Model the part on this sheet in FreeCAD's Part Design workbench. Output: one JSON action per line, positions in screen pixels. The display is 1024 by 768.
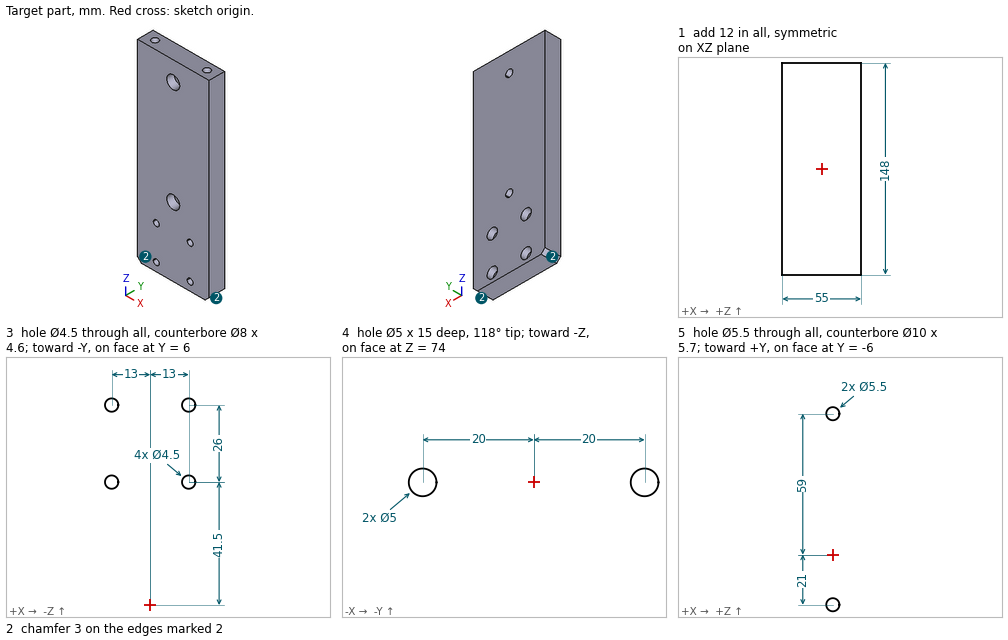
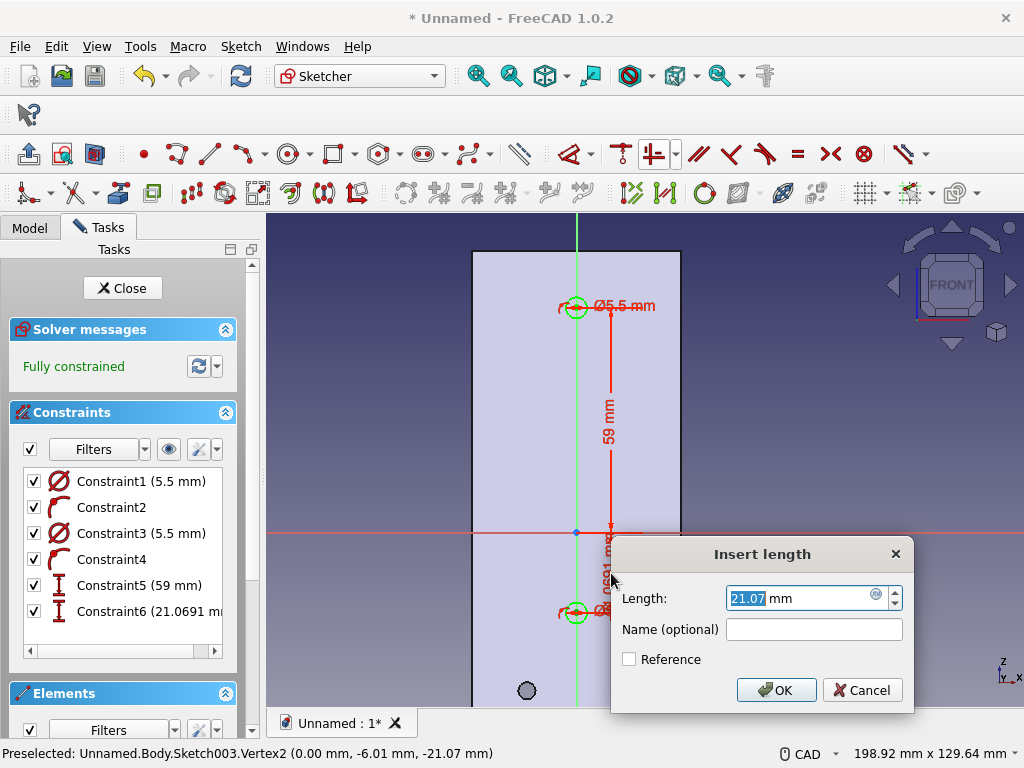
{"action": "type", "text": "21"}
{"action": "key", "text": "Return"}
{"action": "key", "text": "Escape"}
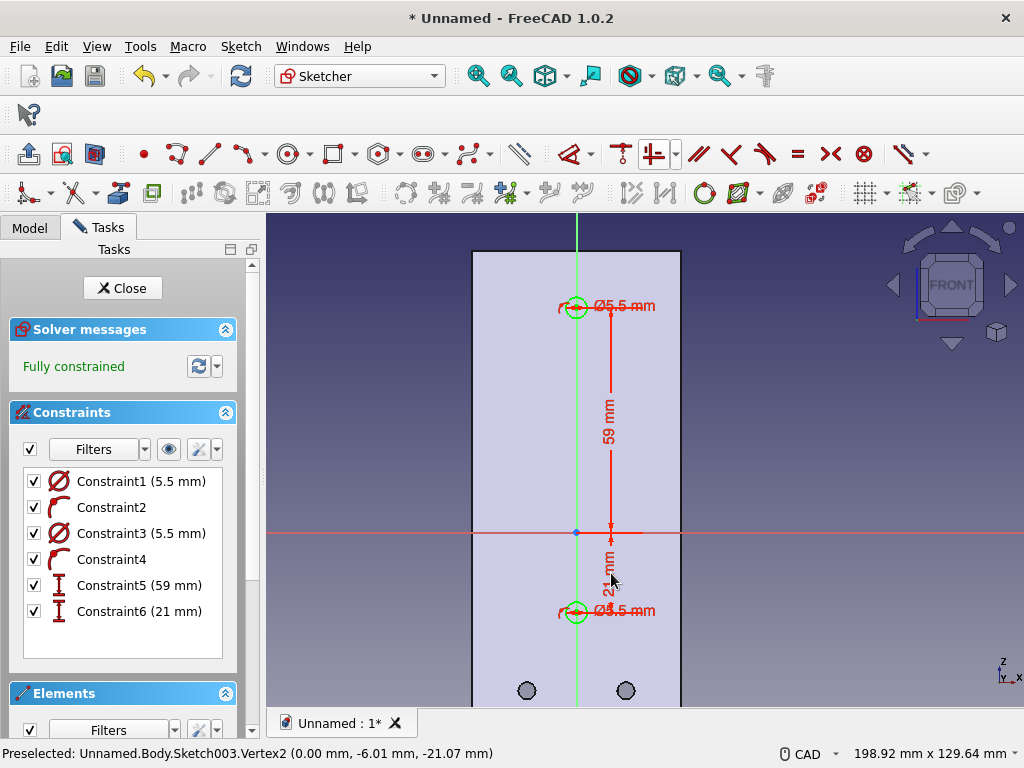
{"action": "left_click", "coordinate": [123, 288]}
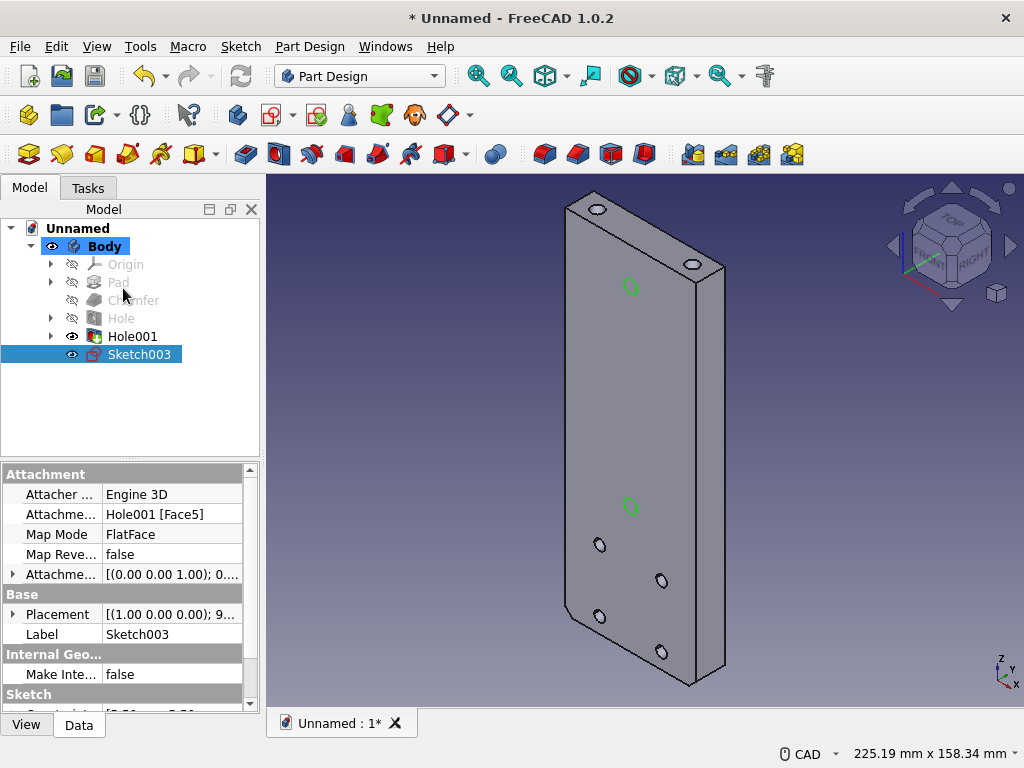
{"action": "left_click", "coordinate": [279, 154]}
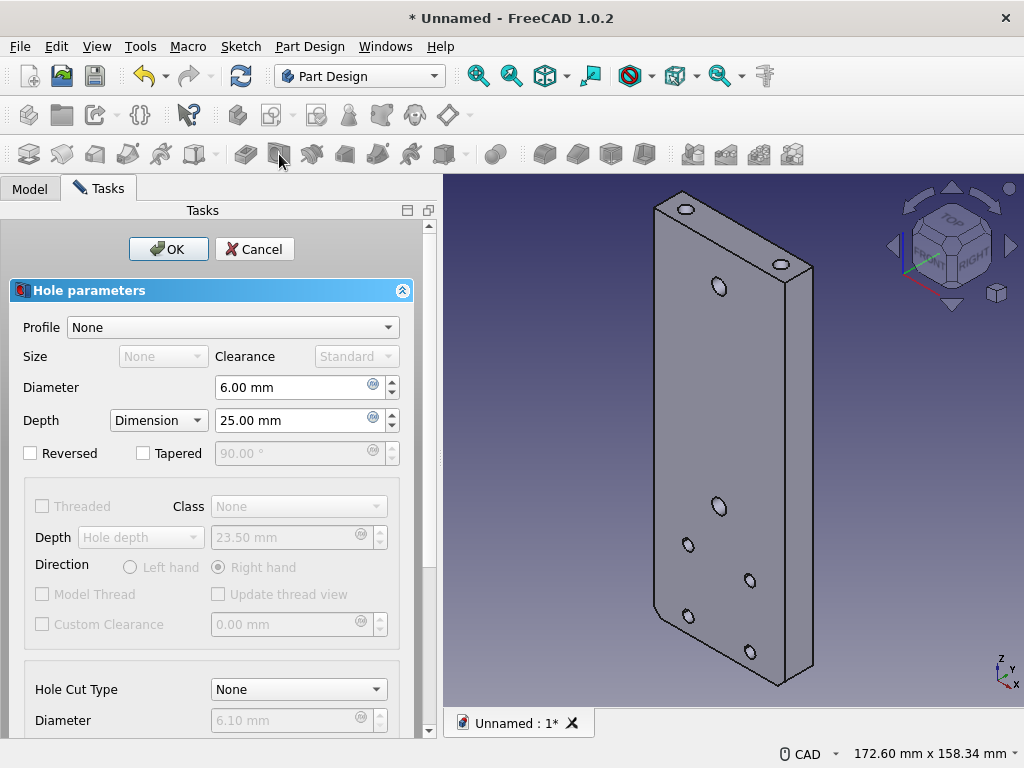
{"action": "triple_click", "coordinate": [300, 388]}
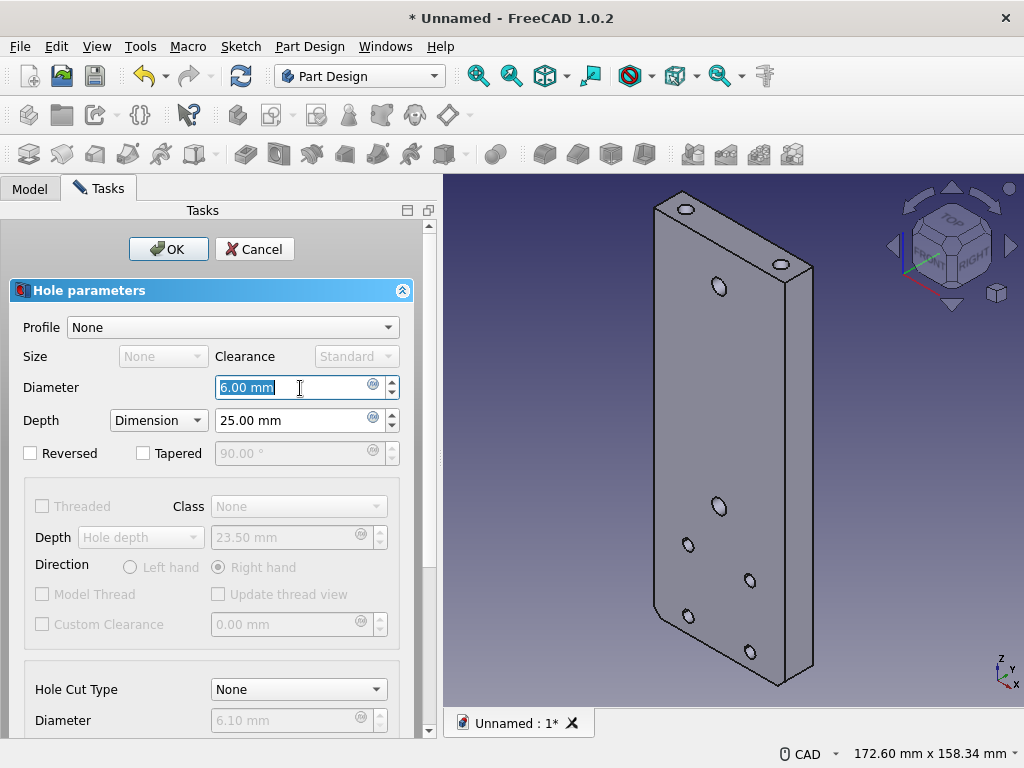
{"action": "type", "text": "5.5"}
{"action": "key", "text": "Tab"}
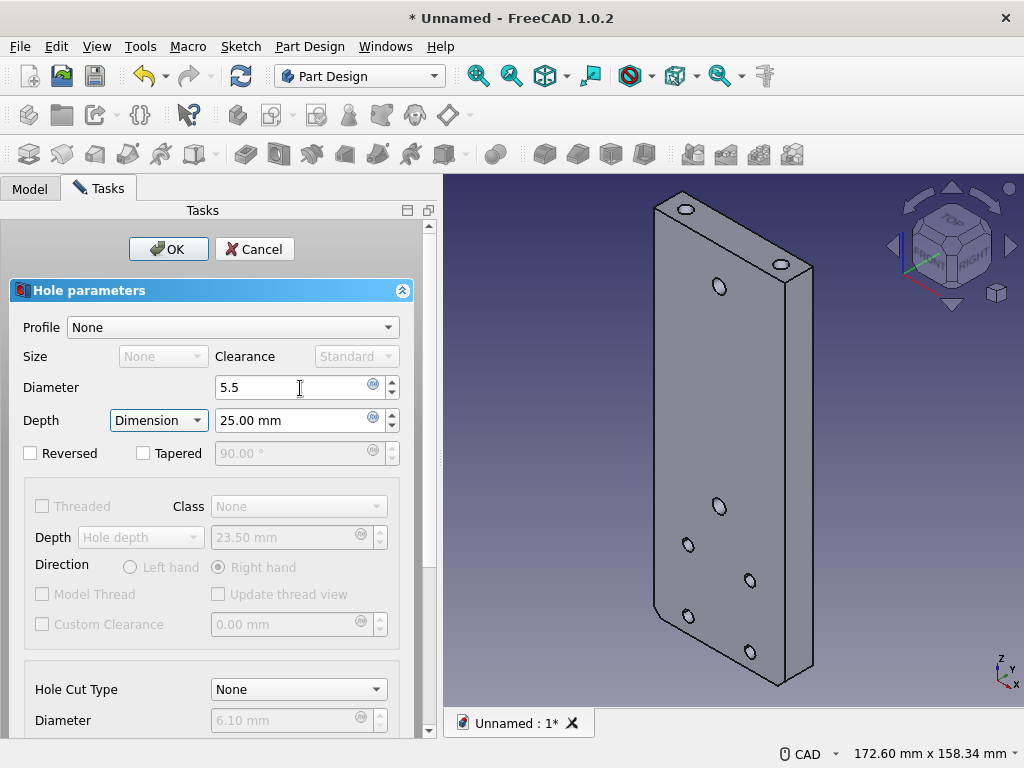
{"action": "left_click", "coordinate": [160, 420]}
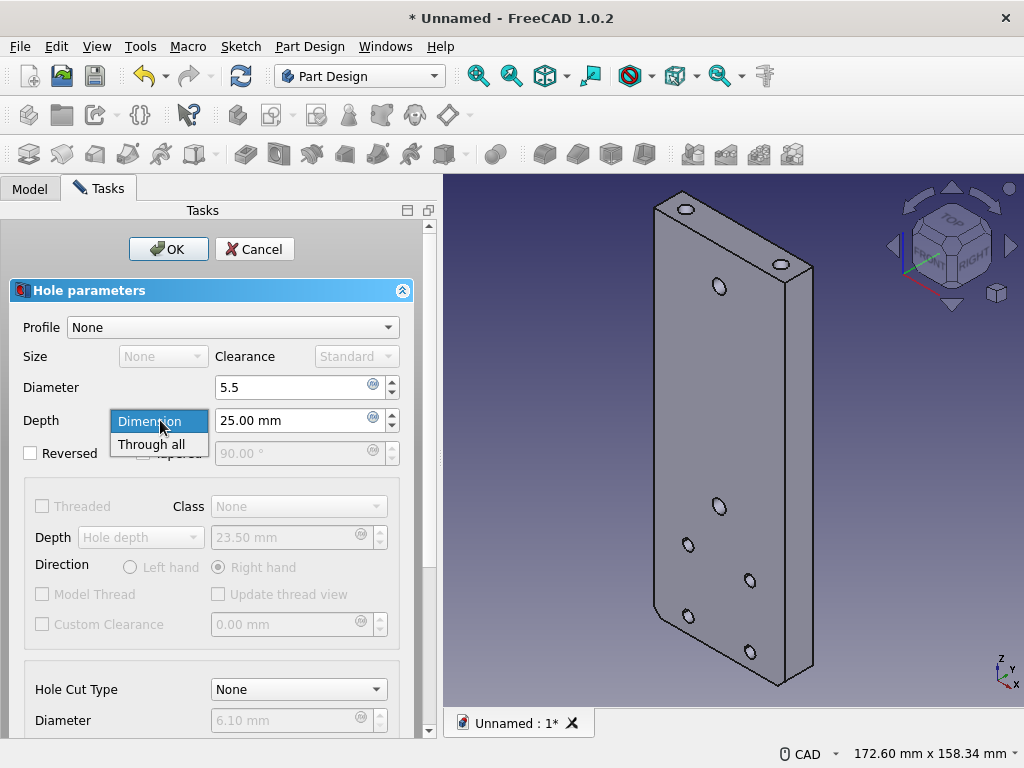
{"action": "left_click", "coordinate": [158, 444]}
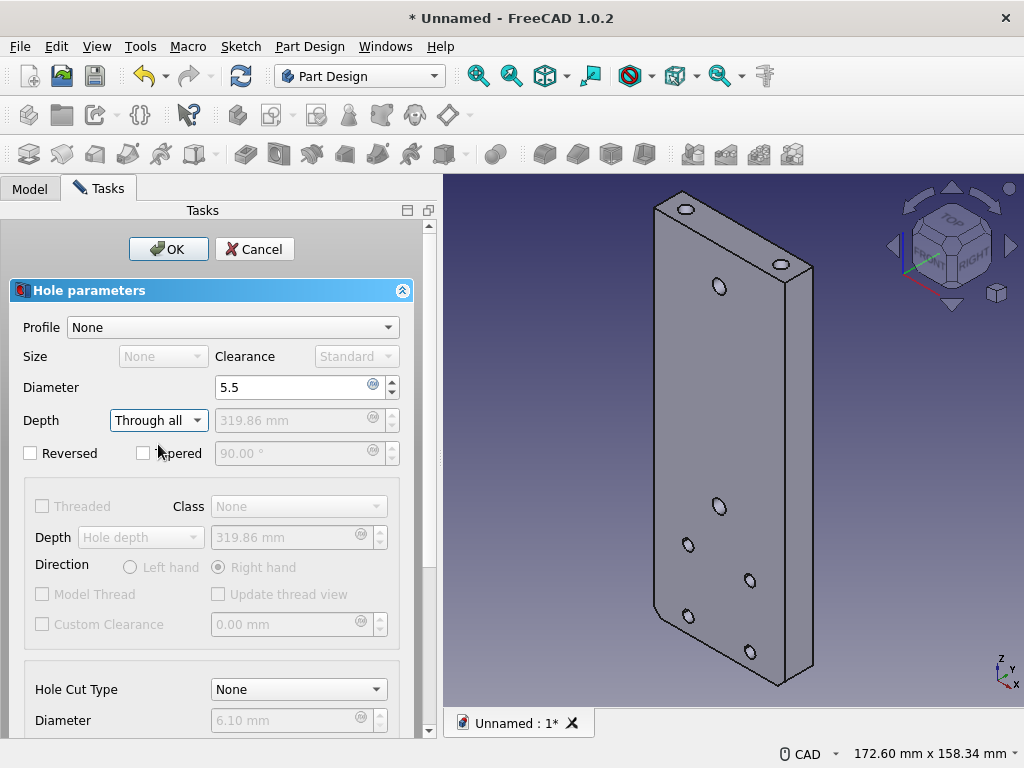
{"action": "left_click", "coordinate": [300, 690]}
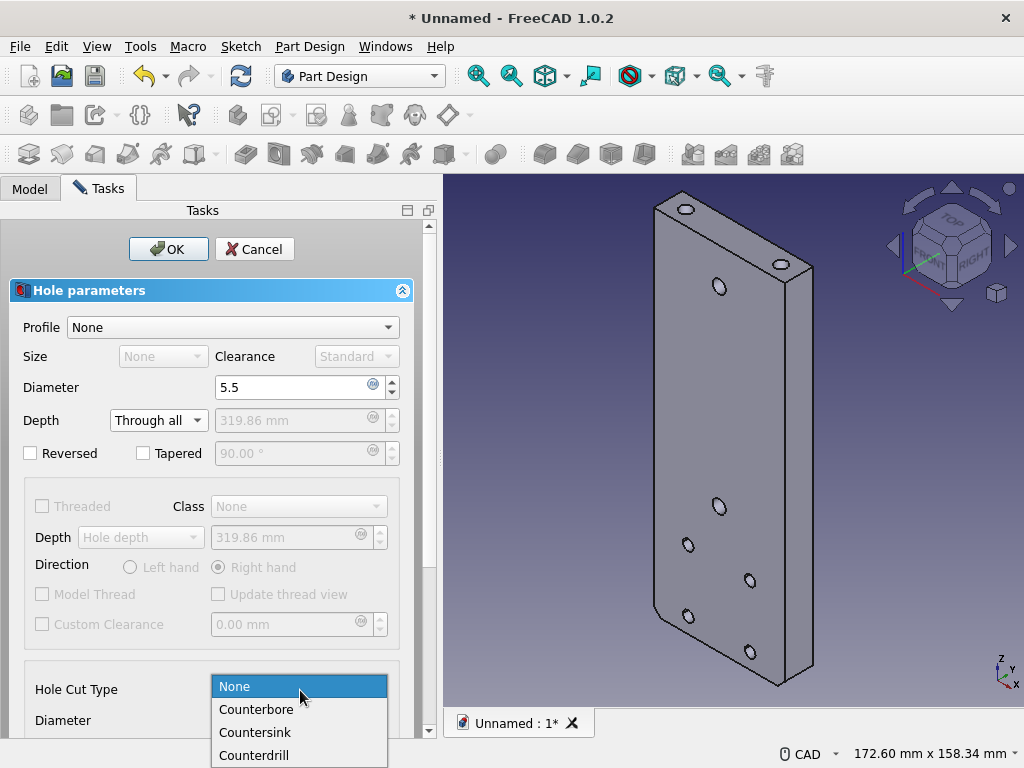
{"action": "left_click", "coordinate": [298, 710]}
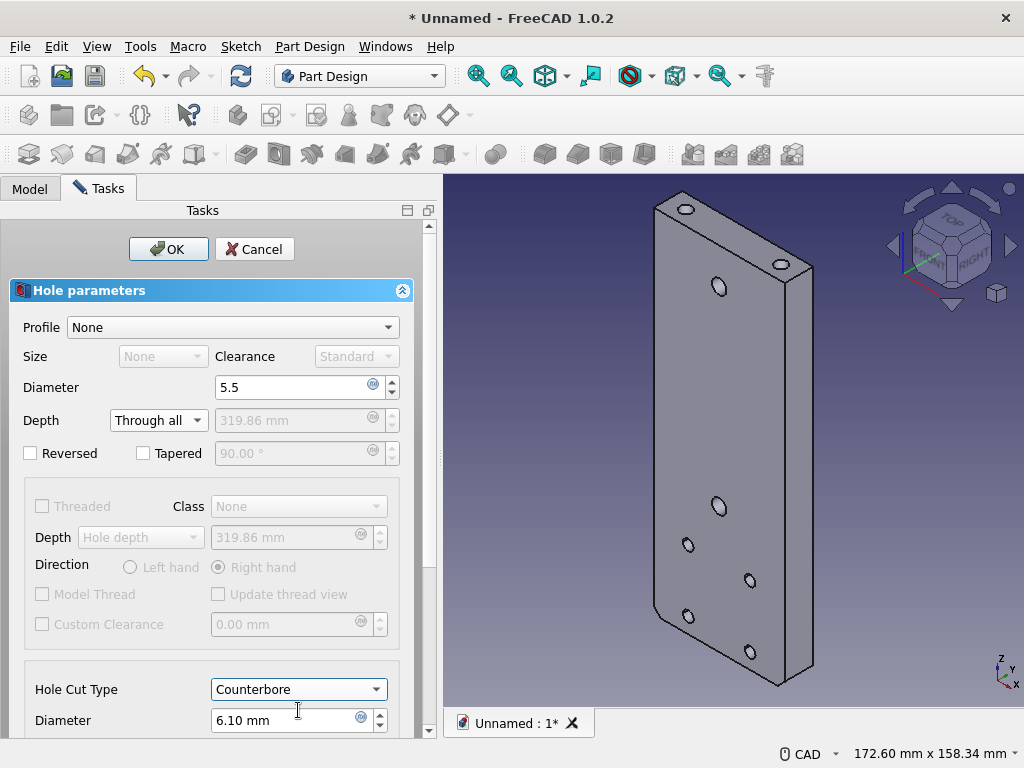
{"action": "triple_click", "coordinate": [292, 720]}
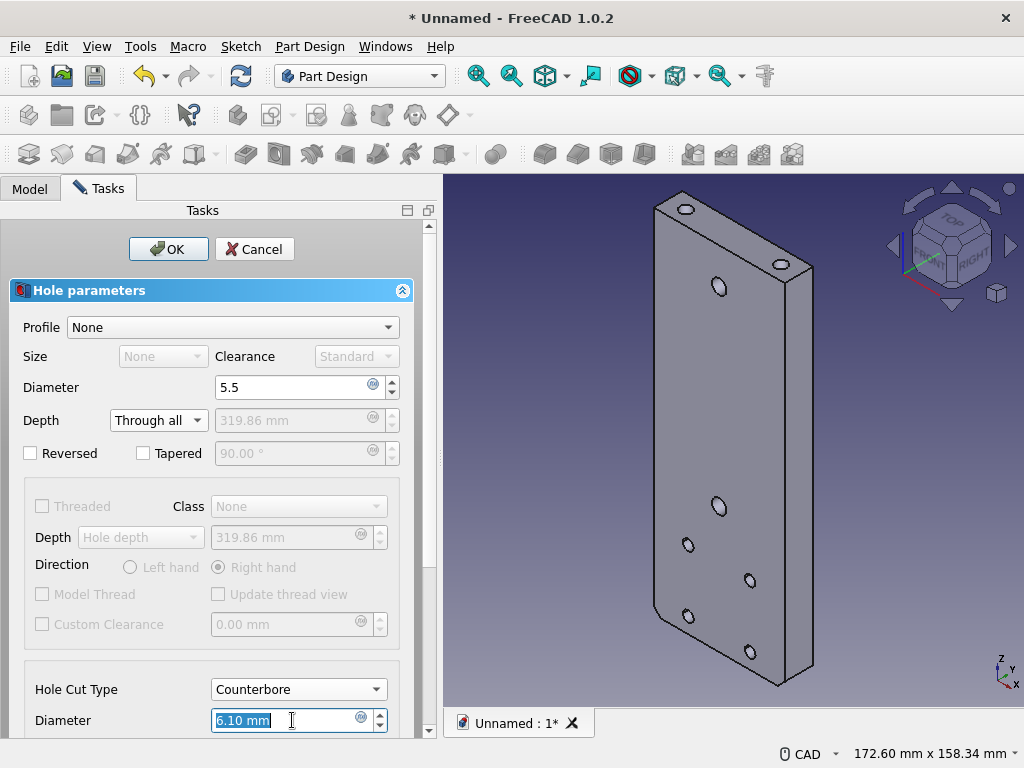
{"action": "type", "text": "10"}
{"action": "key", "text": "Tab"}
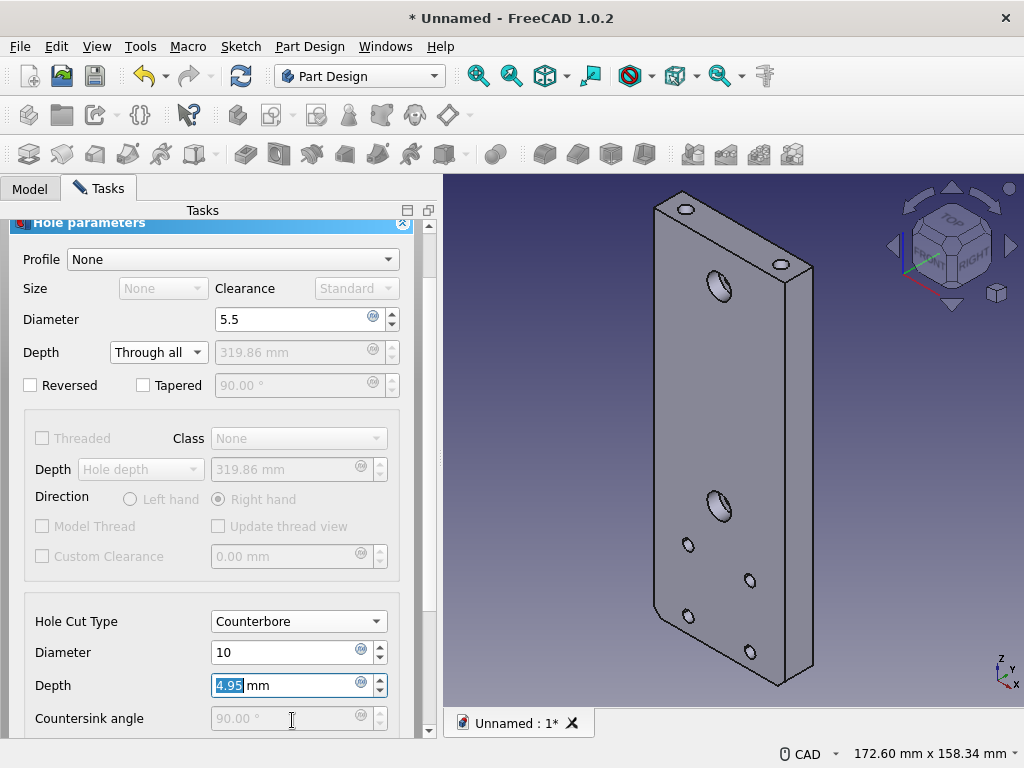
{"action": "type", "text": "5.7"}
{"action": "key", "text": "Tab"}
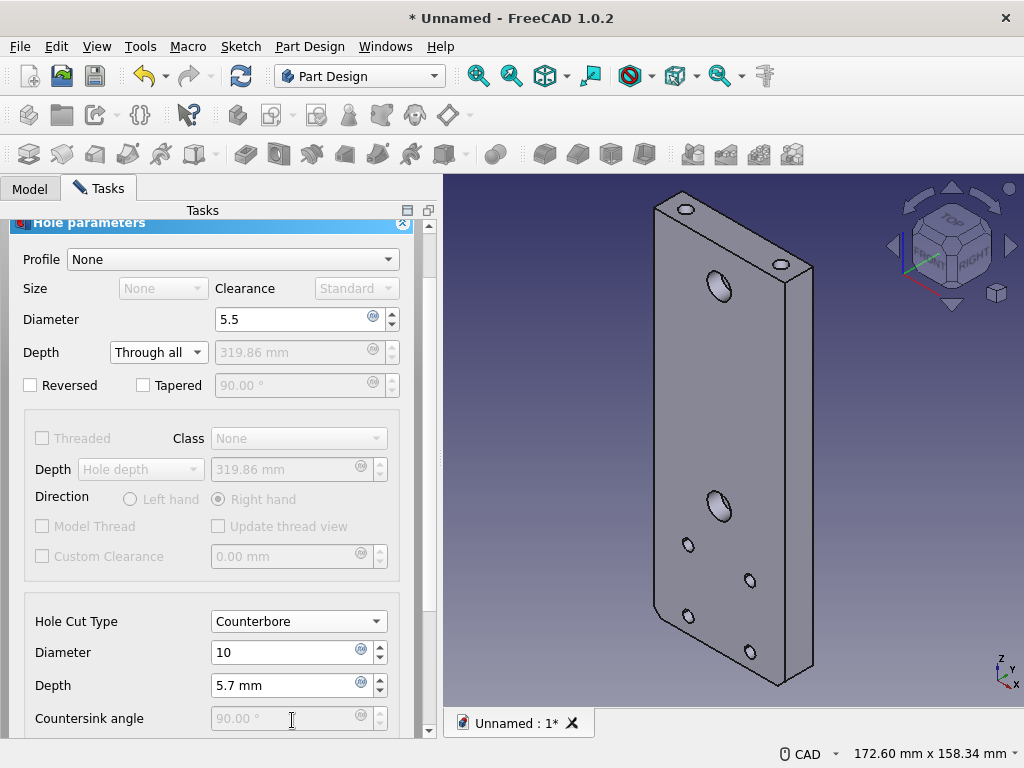
{"action": "scroll", "coordinate": [429, 479], "scroll_direction": "up", "scroll_amount": 2}